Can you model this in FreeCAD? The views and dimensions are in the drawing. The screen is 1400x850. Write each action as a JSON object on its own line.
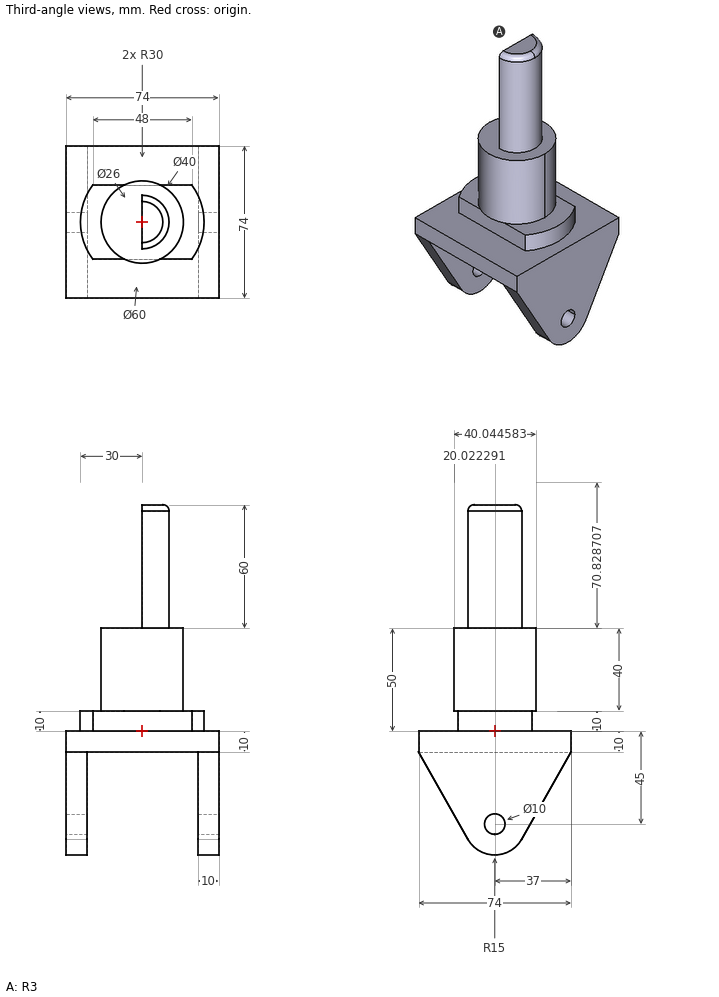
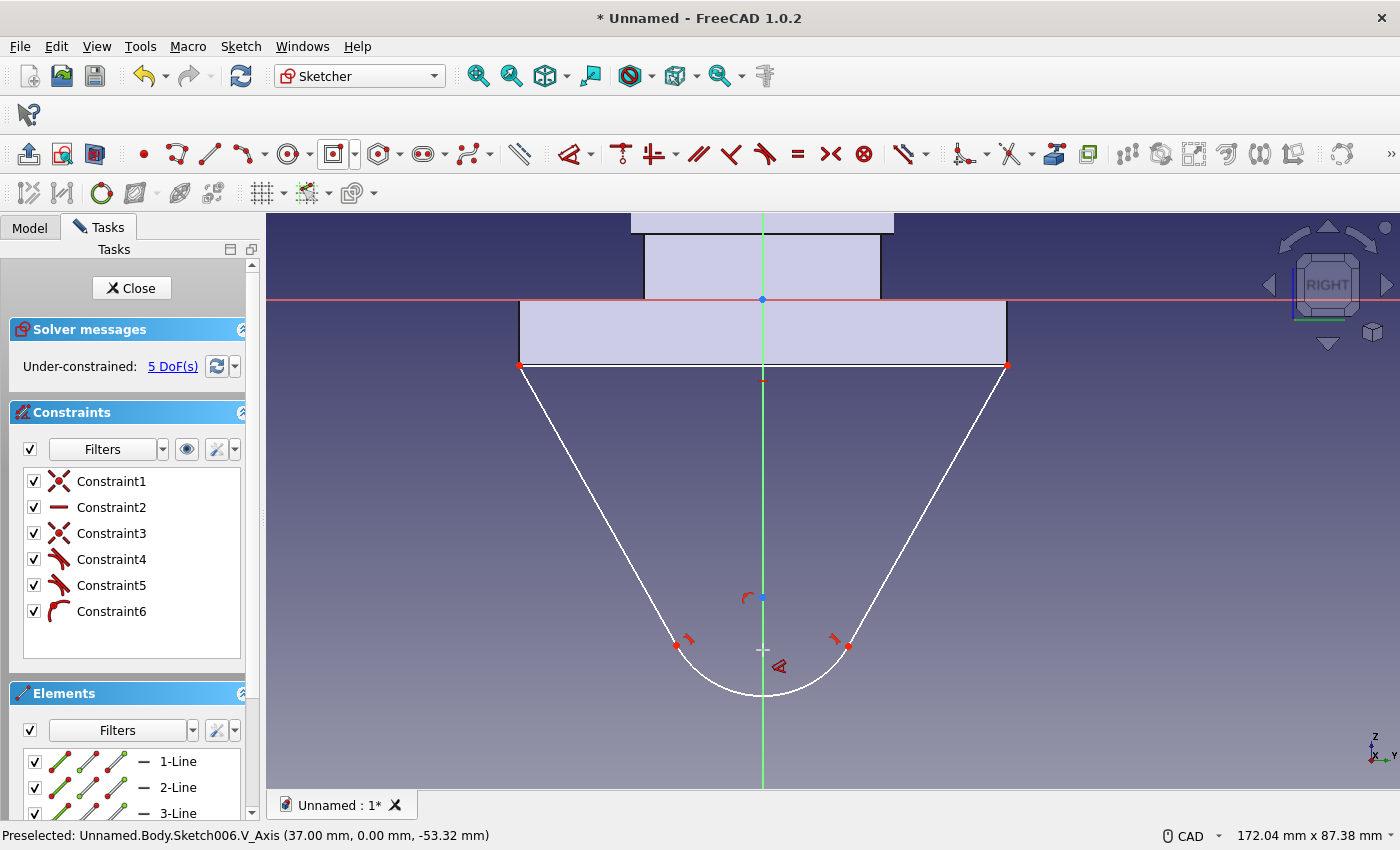
{"action": "left_click", "coordinate": [722, 687]}
{"action": "left_click", "coordinate": [709, 716]}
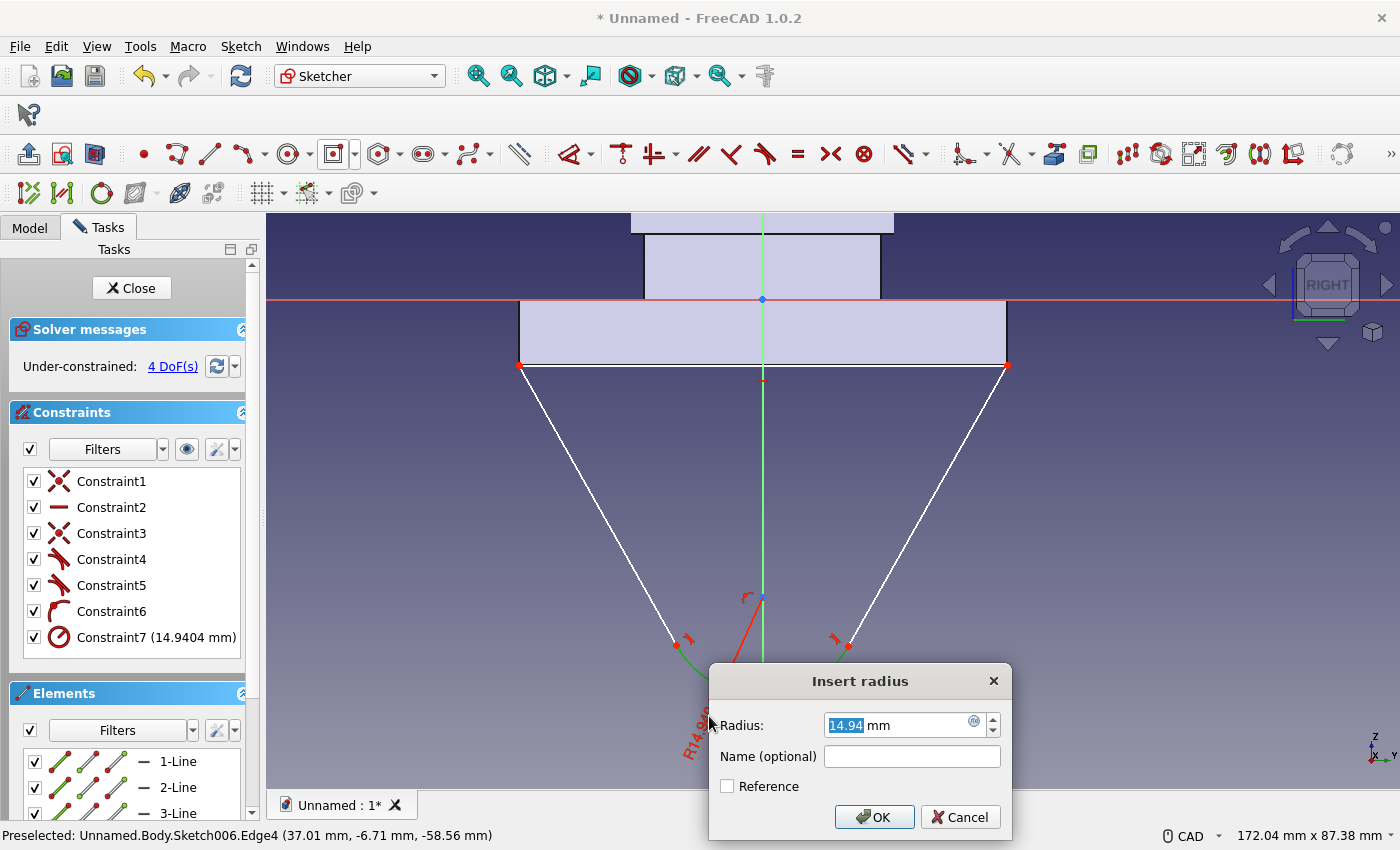
{"action": "type", "text": "15"}
{"action": "key", "text": "Return"}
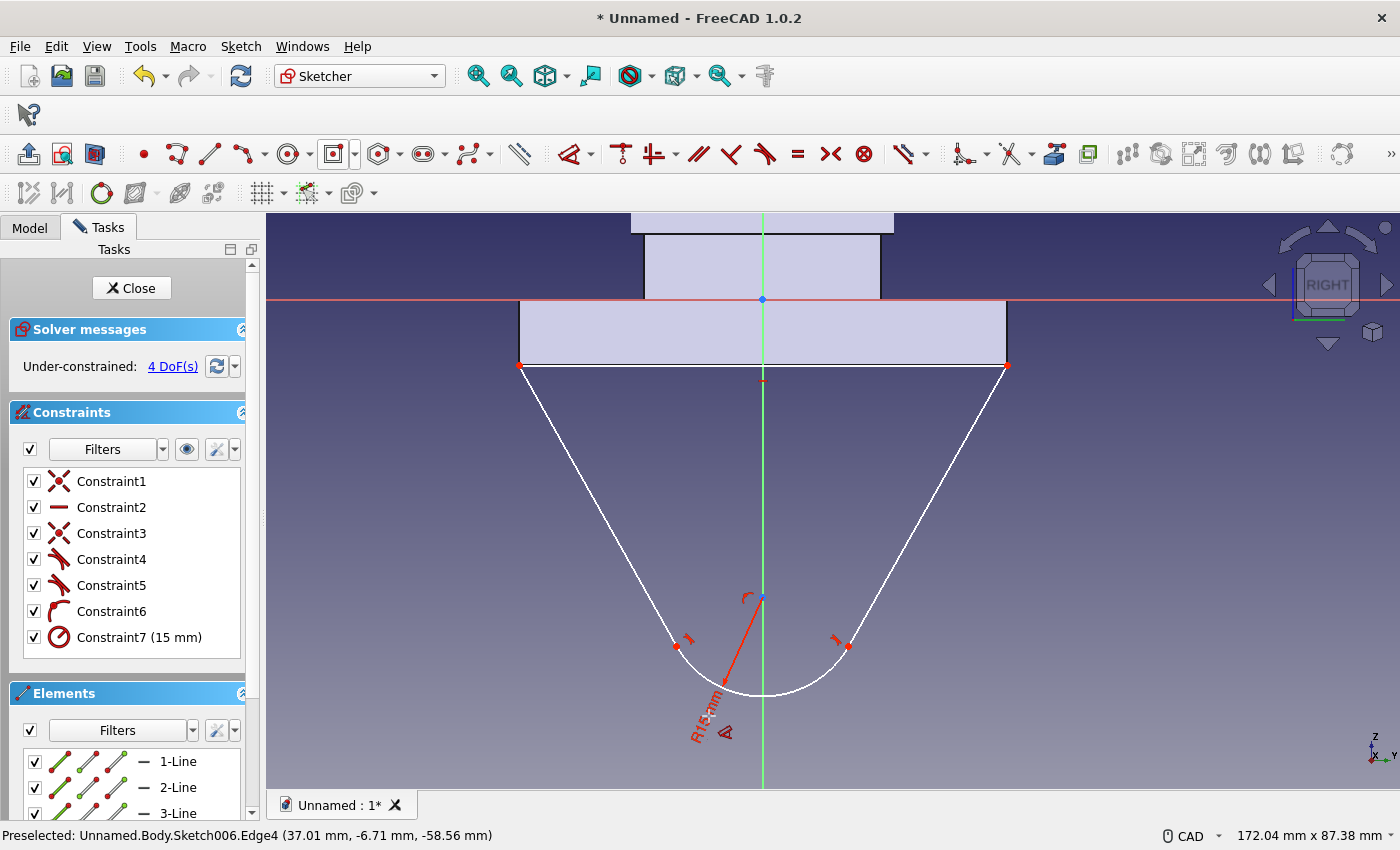
{"action": "left_click", "coordinate": [861, 366]}
{"action": "left_click", "coordinate": [651, 332]}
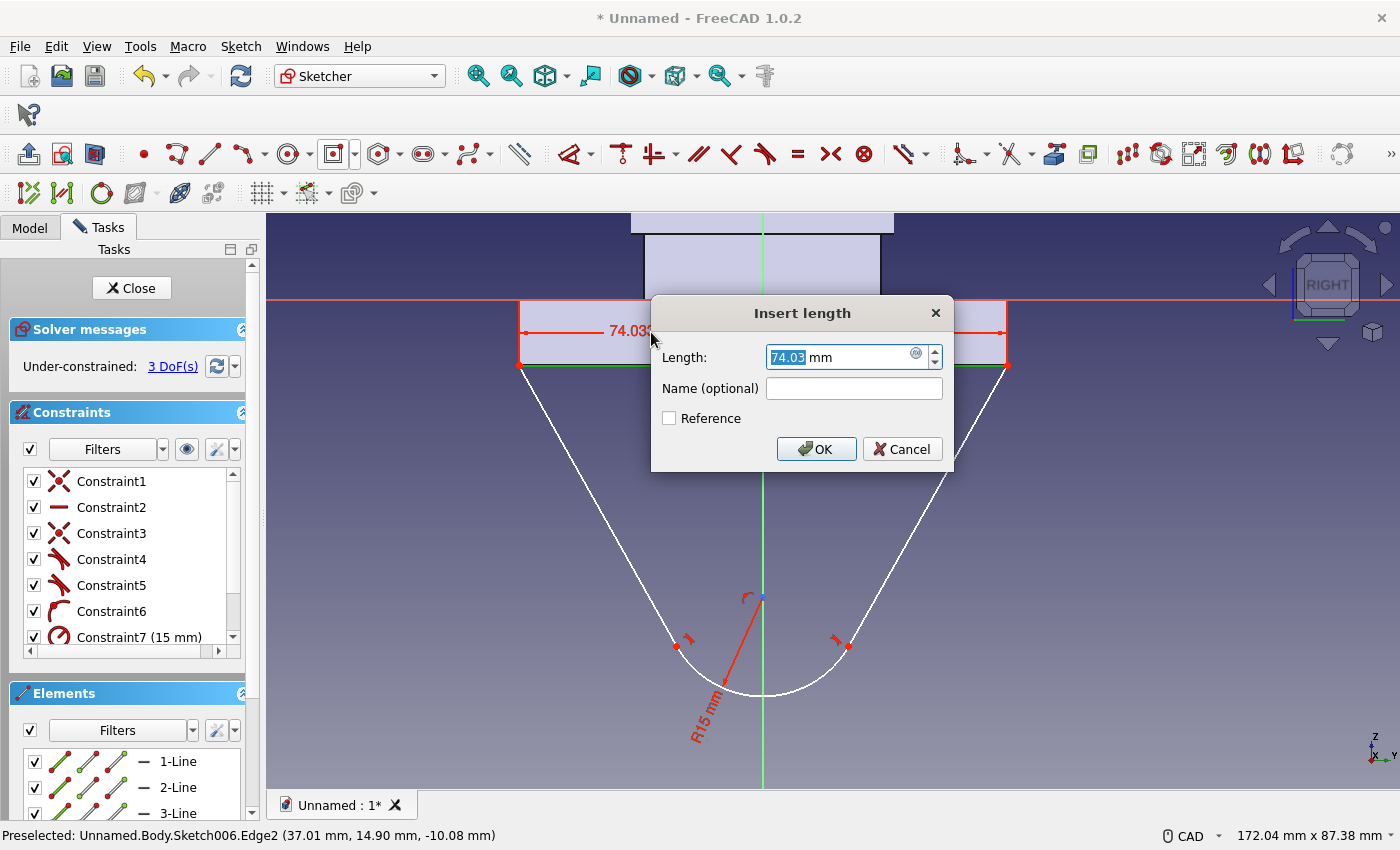
{"action": "type", "text": "74"}
{"action": "key", "text": "Return"}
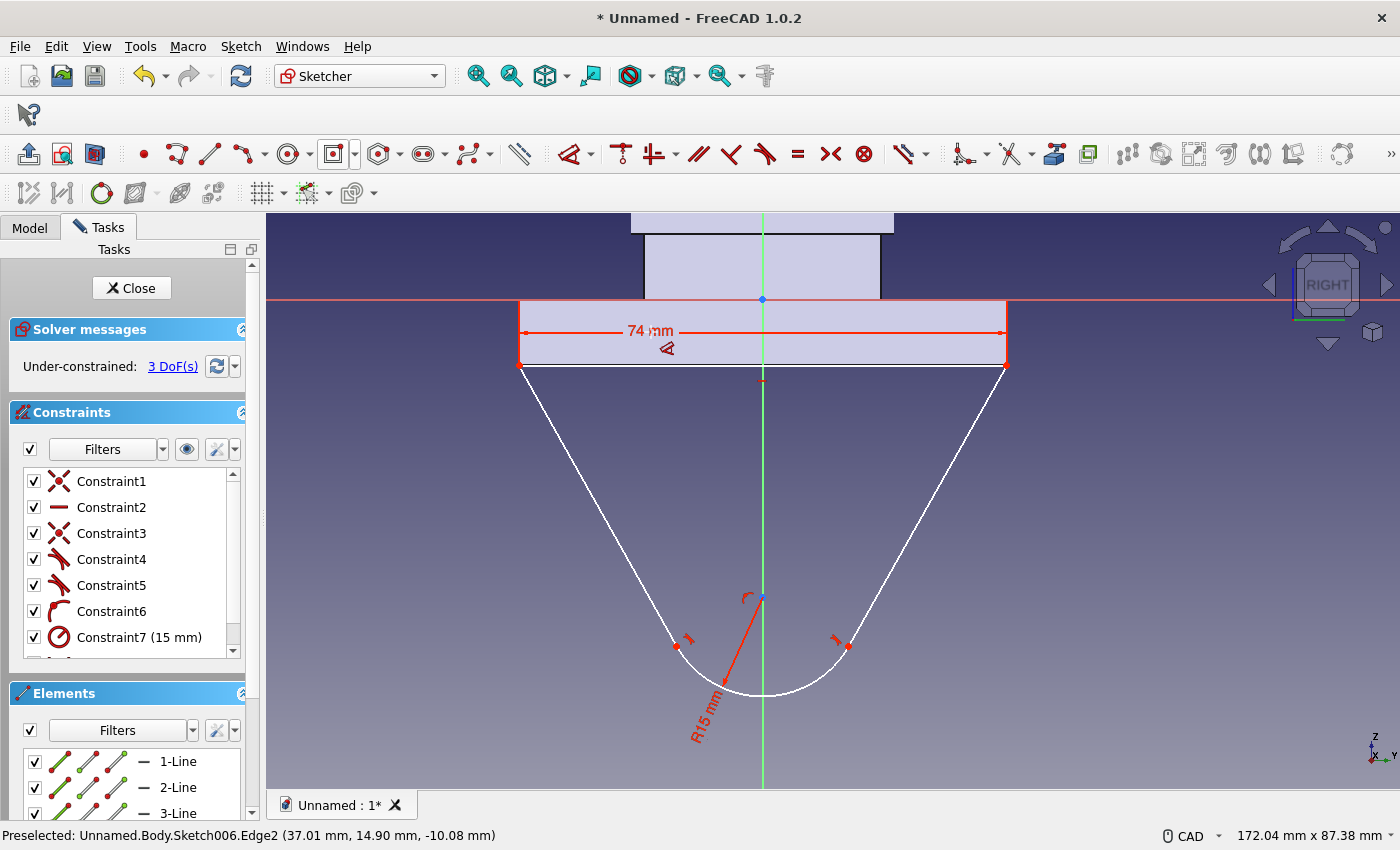
{"action": "left_click", "coordinate": [1007, 366]}
{"action": "left_click", "coordinate": [885, 266]}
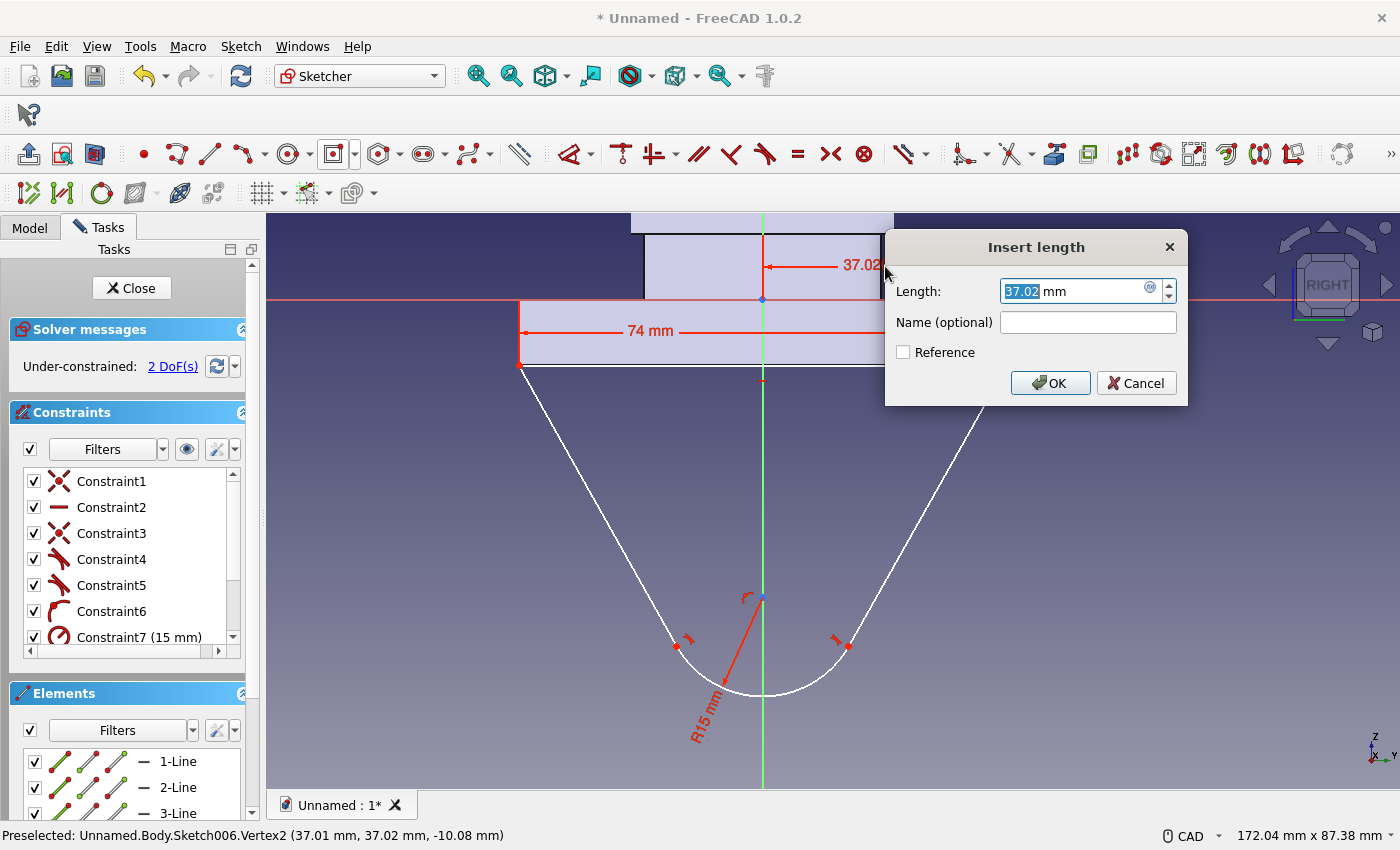
{"action": "type", "text": "37"}
{"action": "key", "text": "Return"}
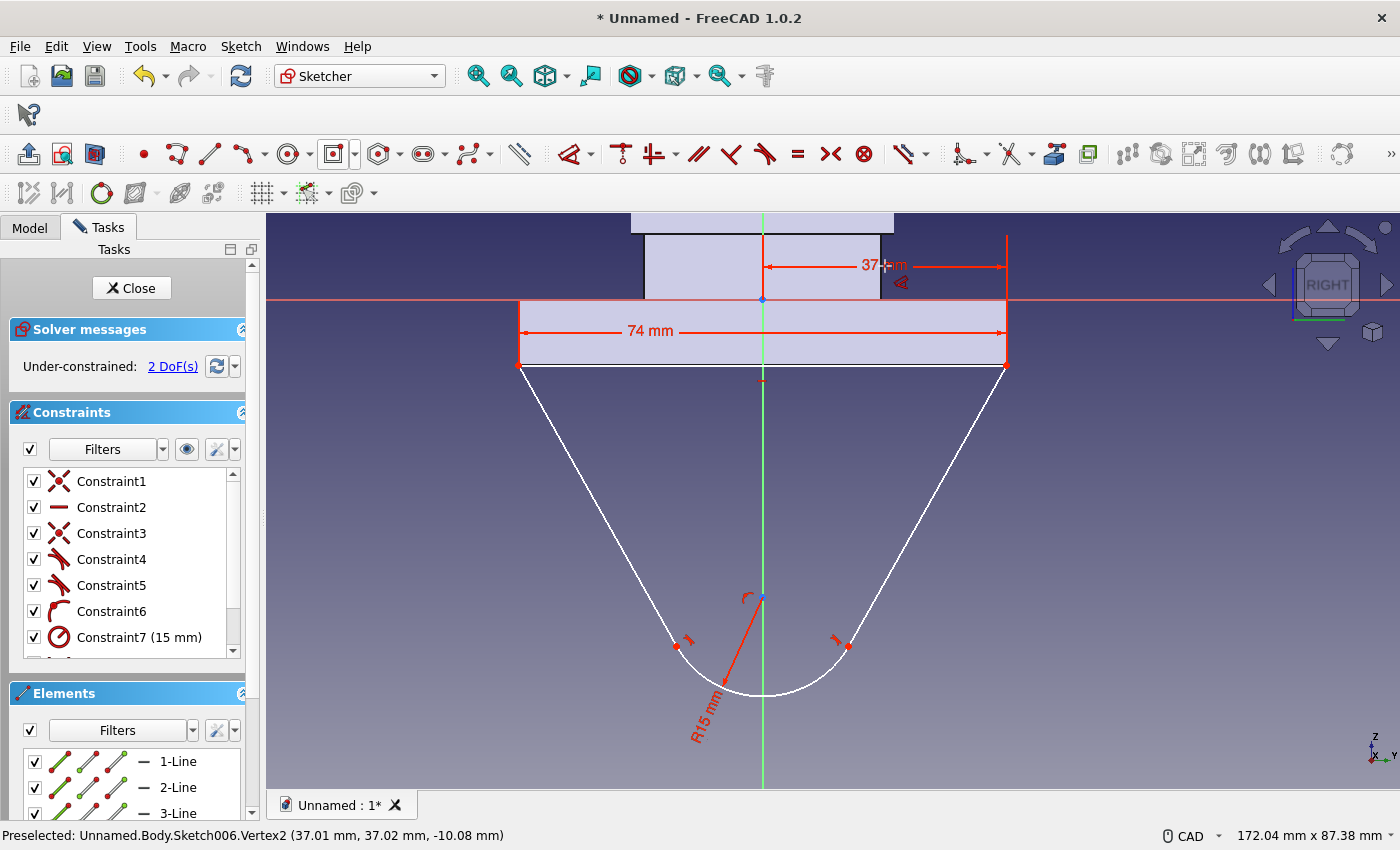
{"action": "left_click", "coordinate": [1007, 366]}
{"action": "left_click", "coordinate": [1041, 333]}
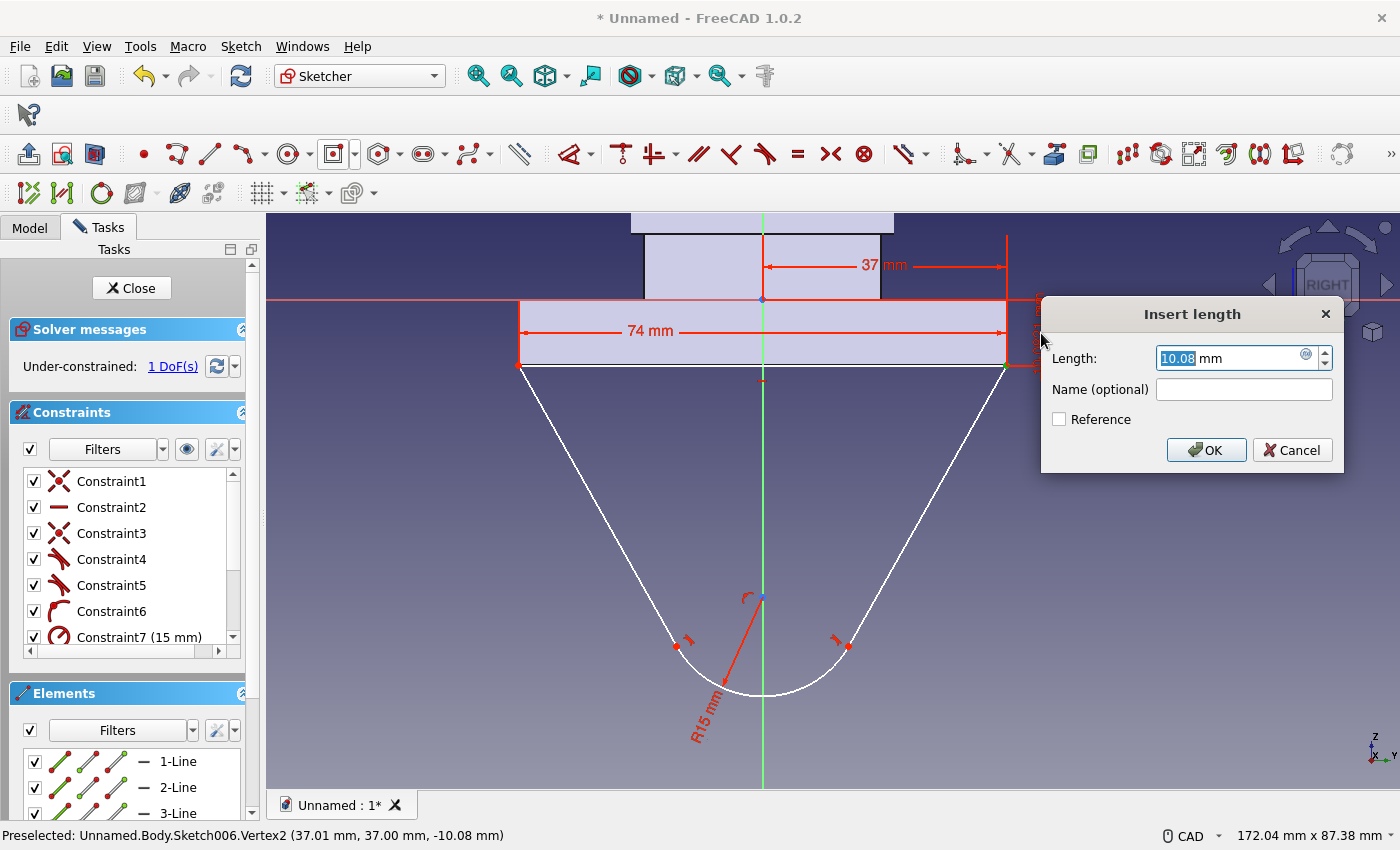
{"action": "type", "text": "10"}
{"action": "key", "text": "Return"}